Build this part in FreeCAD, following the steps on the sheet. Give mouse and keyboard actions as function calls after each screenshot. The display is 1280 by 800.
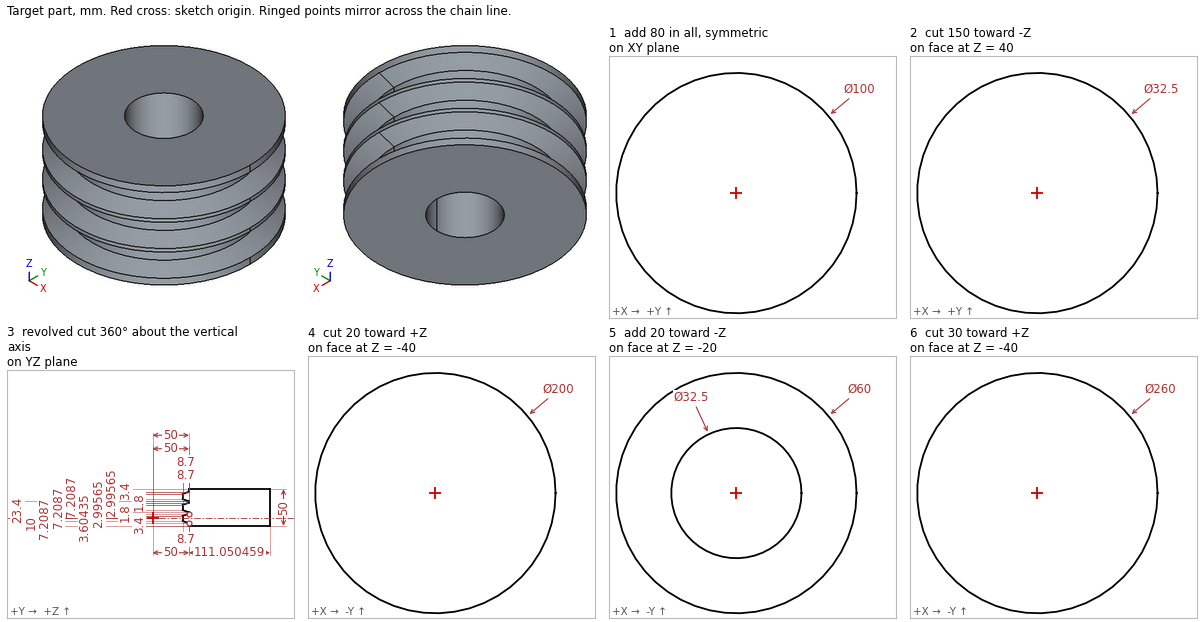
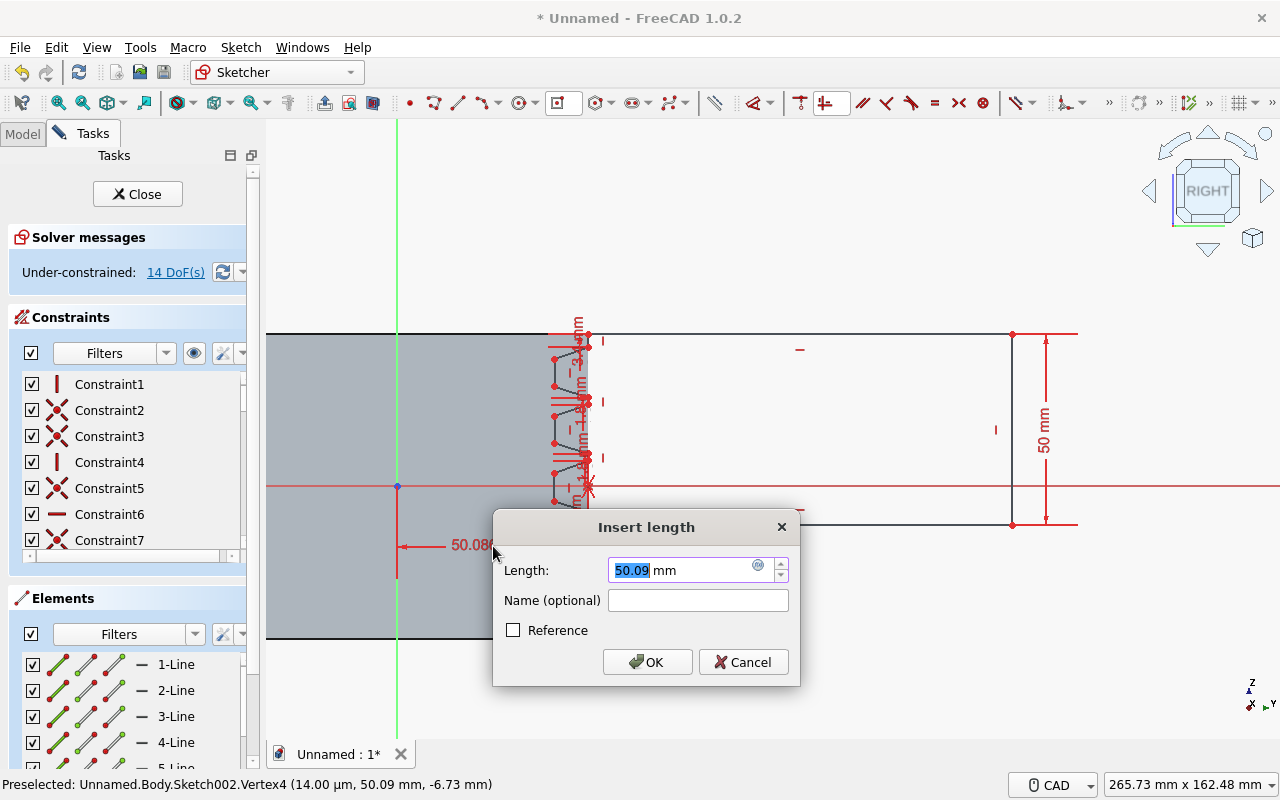
text(50)
key(Return)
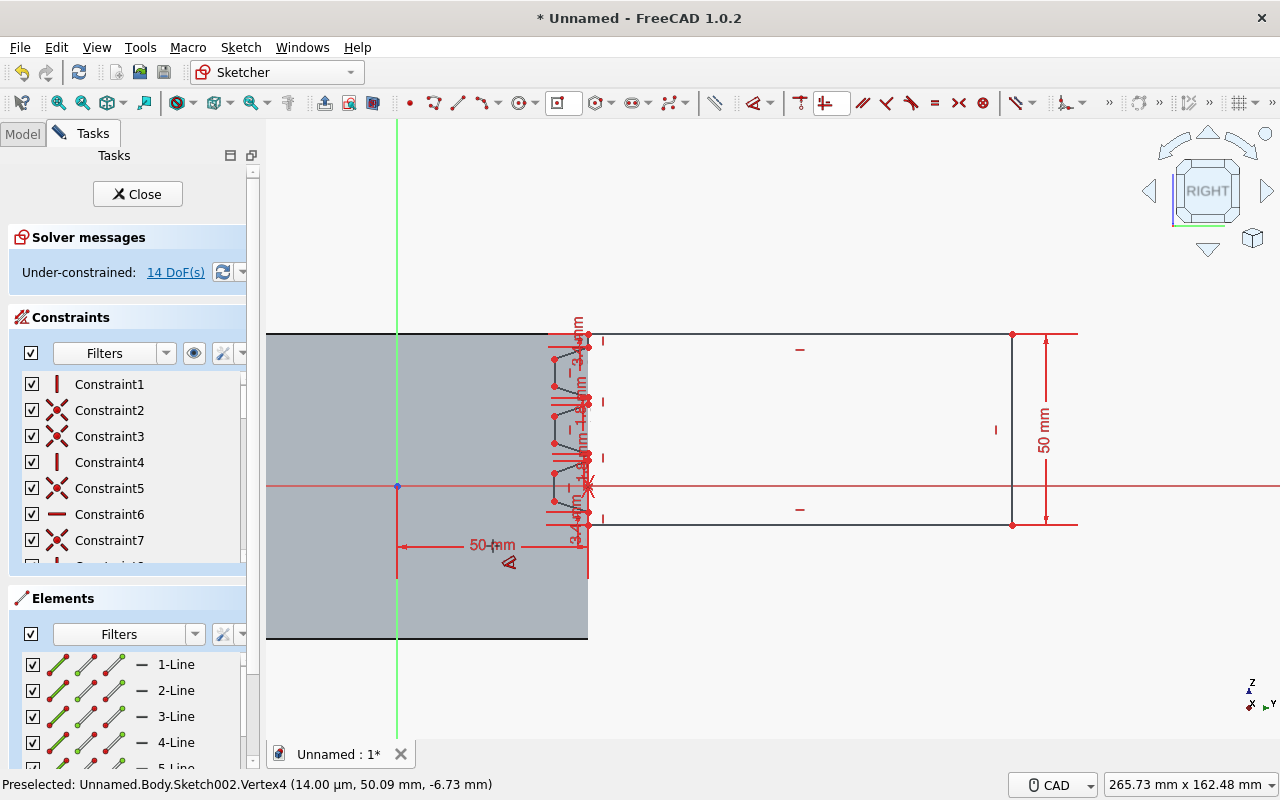
click(588, 525)
click(363, 506)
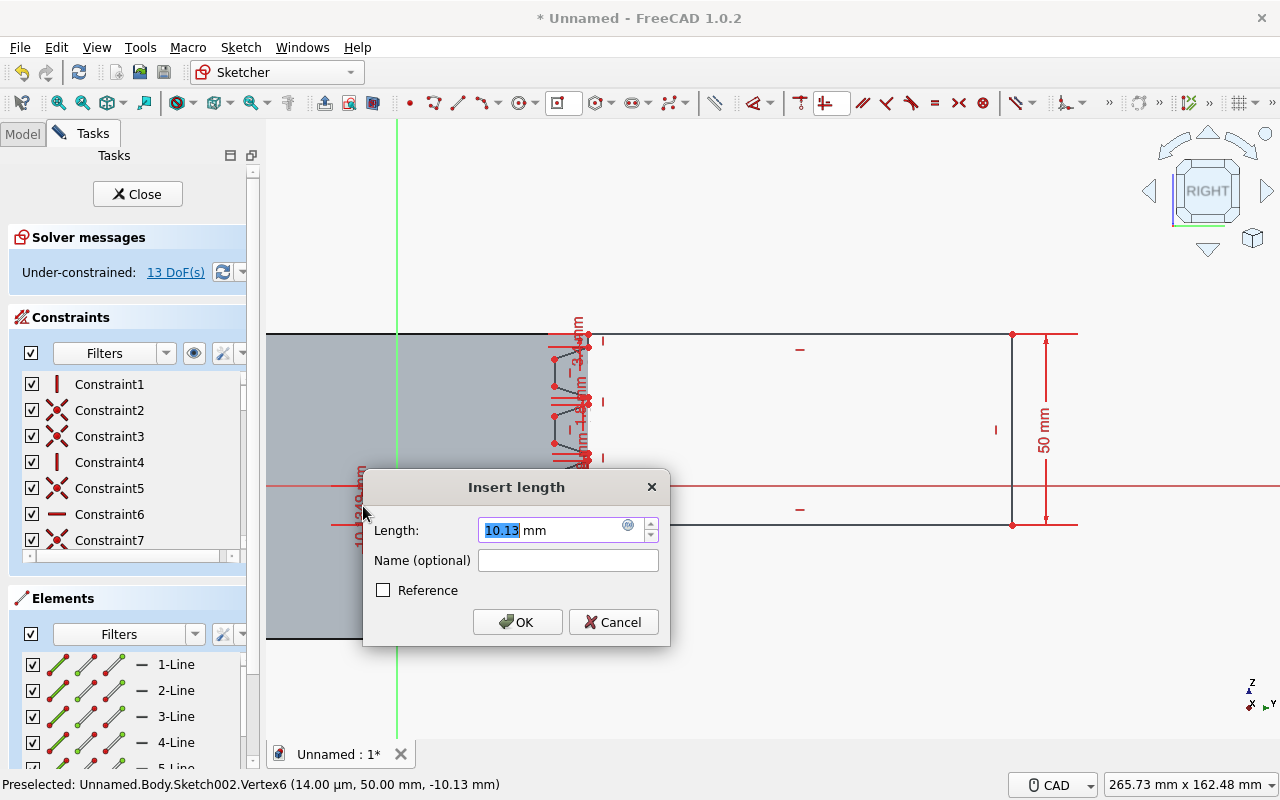
text(10)
key(Return)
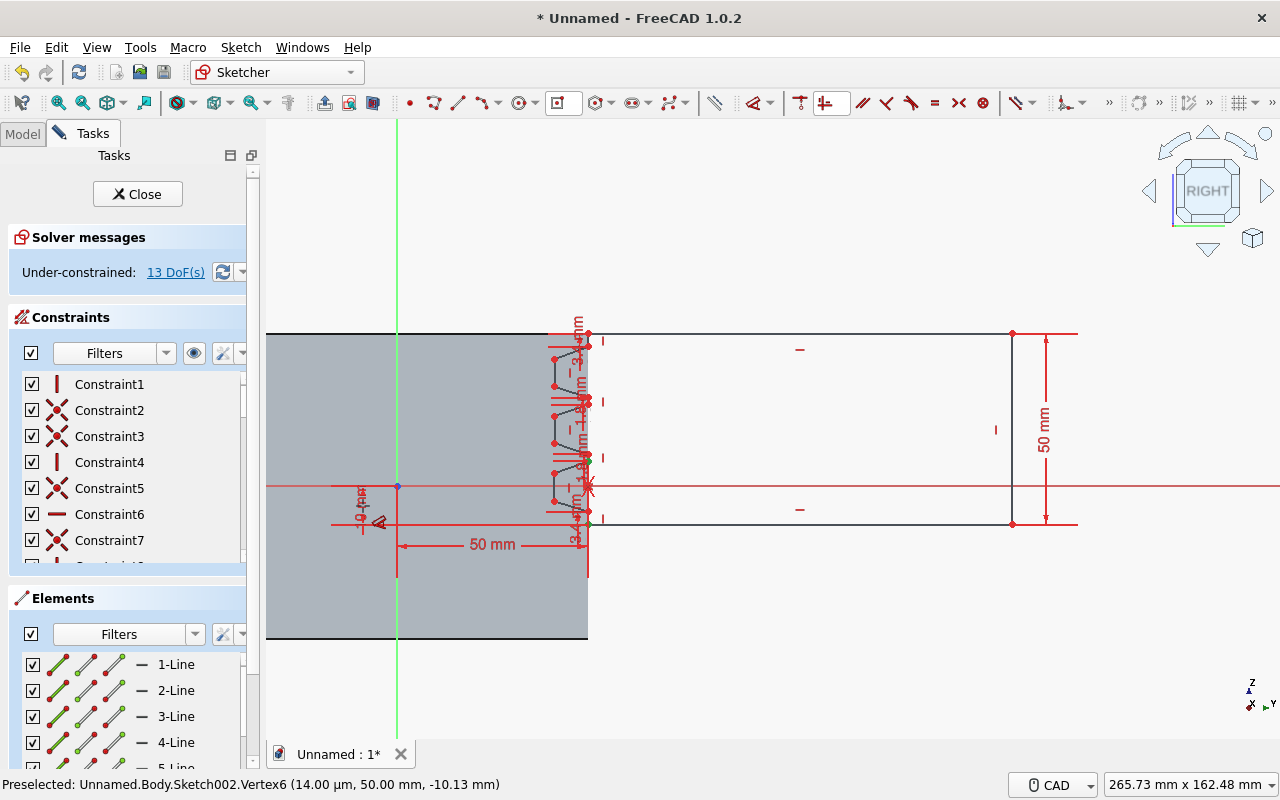
click(588, 334)
click(493, 300)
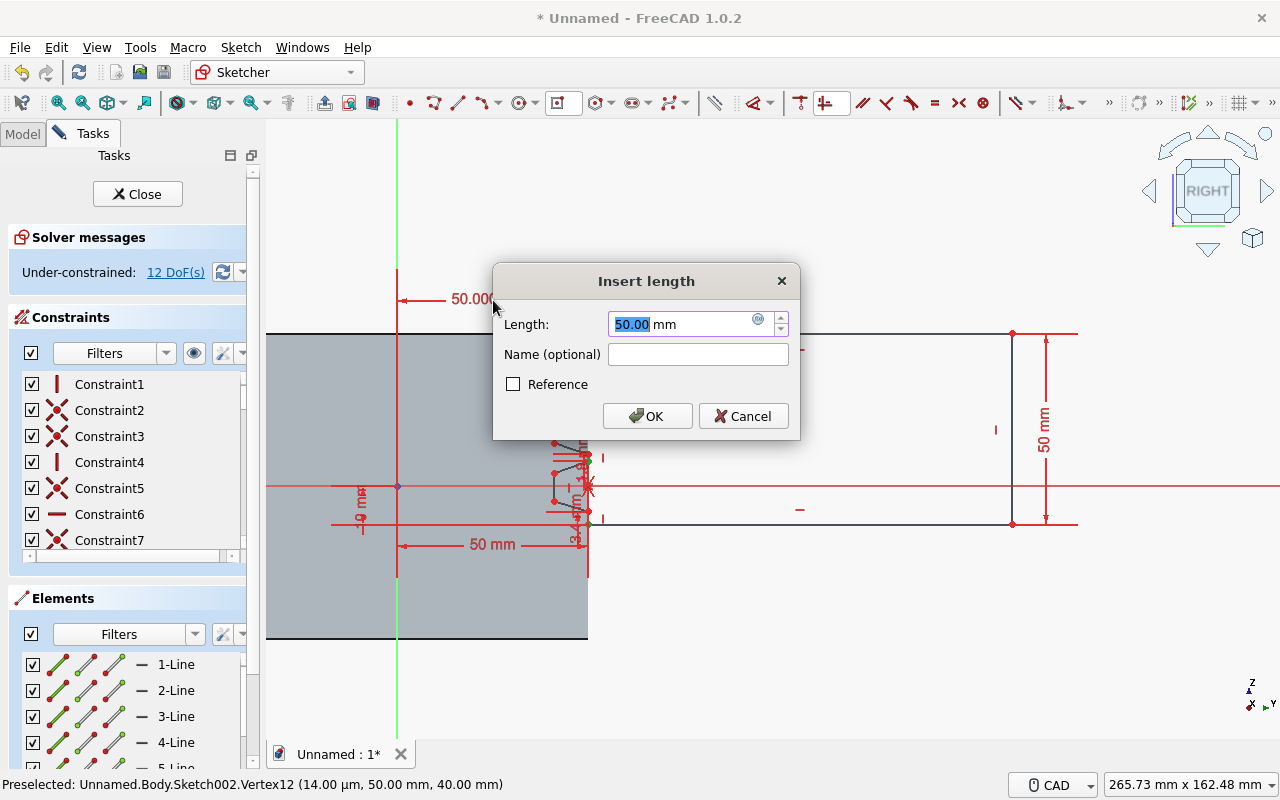
text(50)
key(Return)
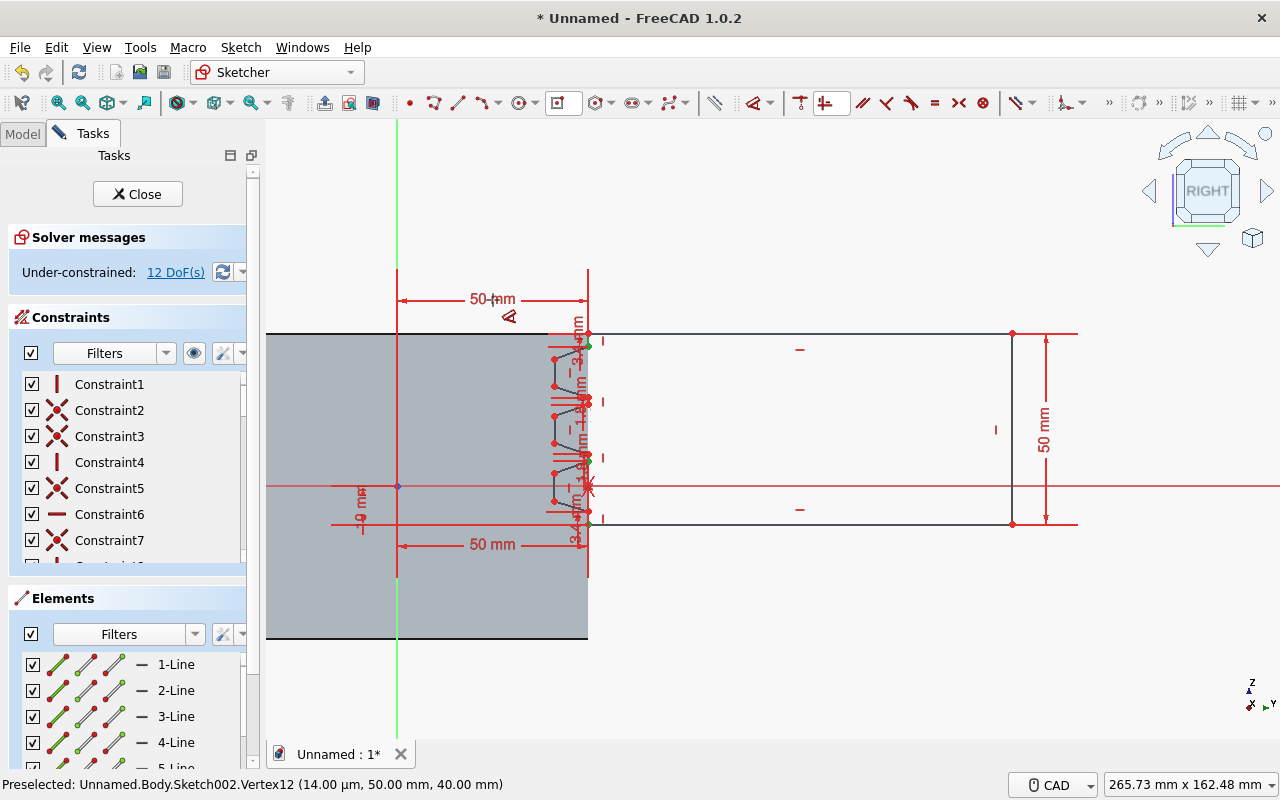
scroll(588, 398, up, 3)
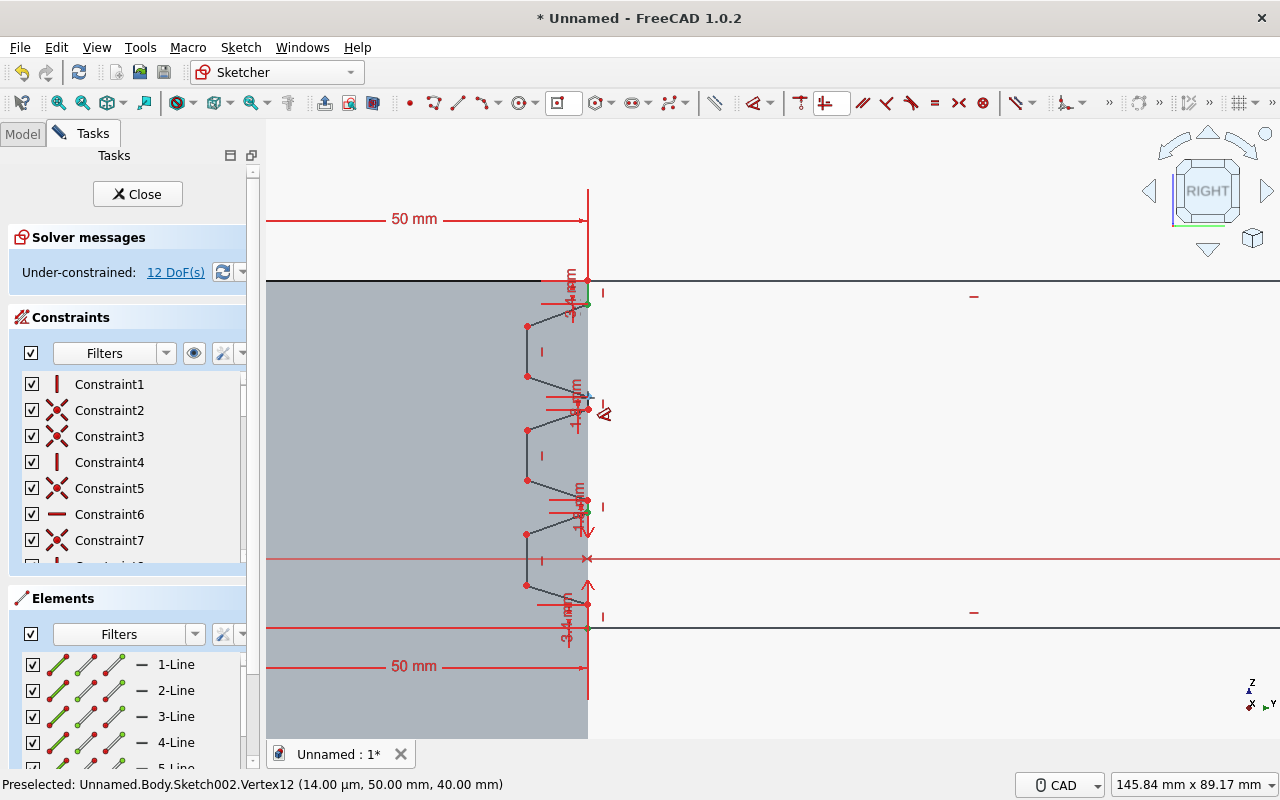
click(588, 397)
click(441, 593)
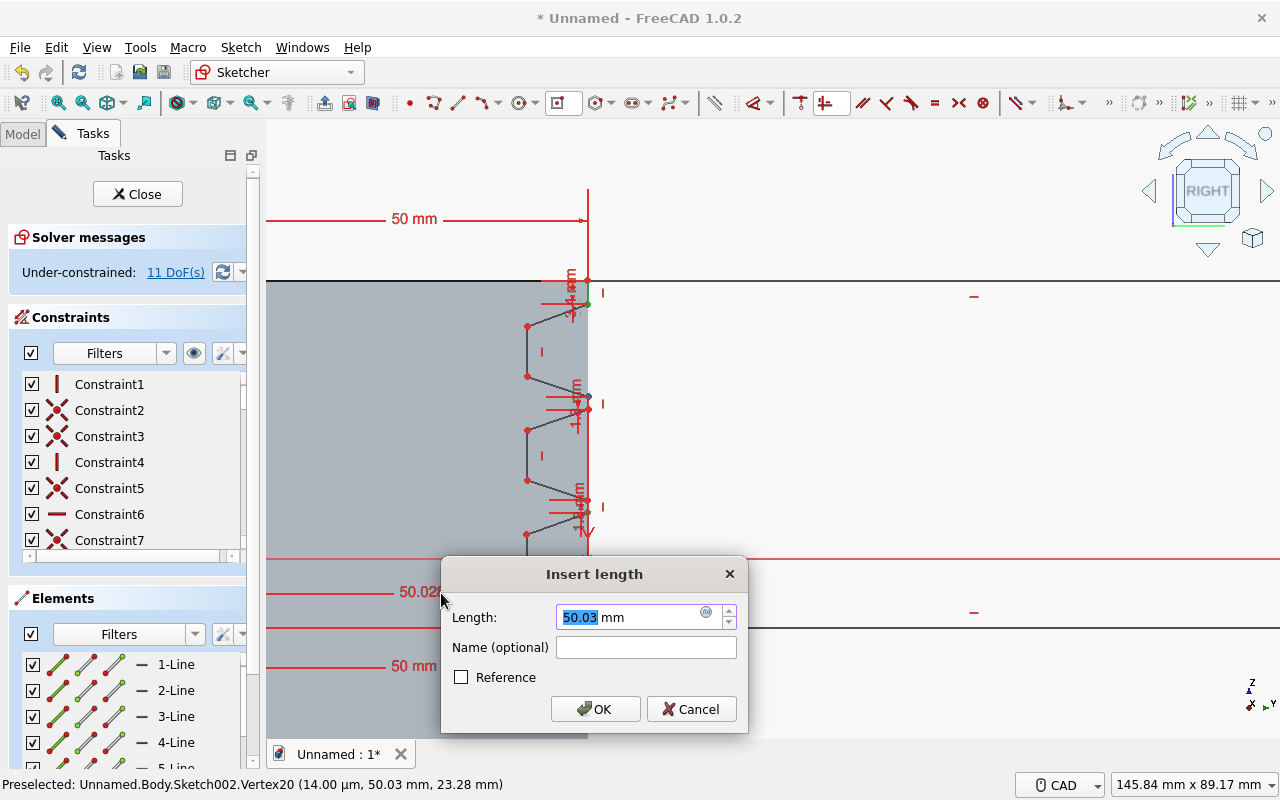
text(50)
key(Return)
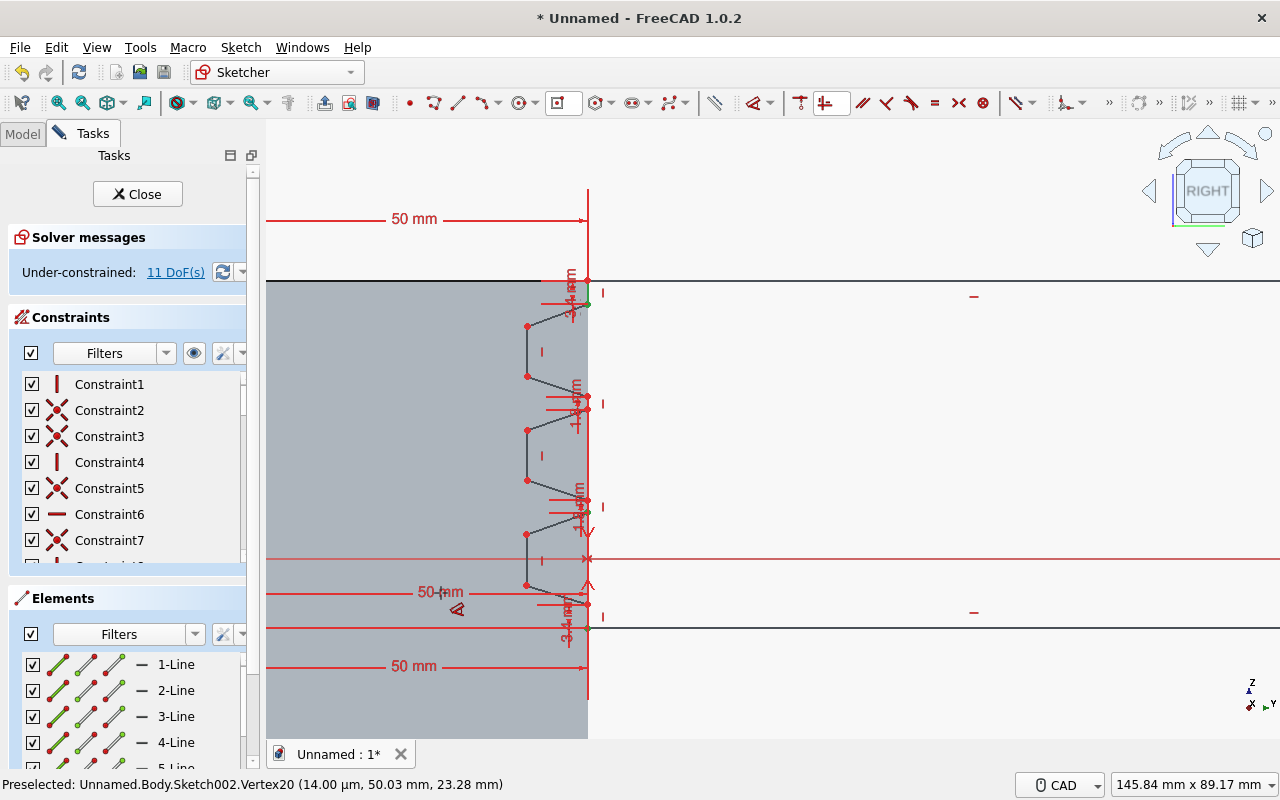
click(545, 592)
click(557, 639)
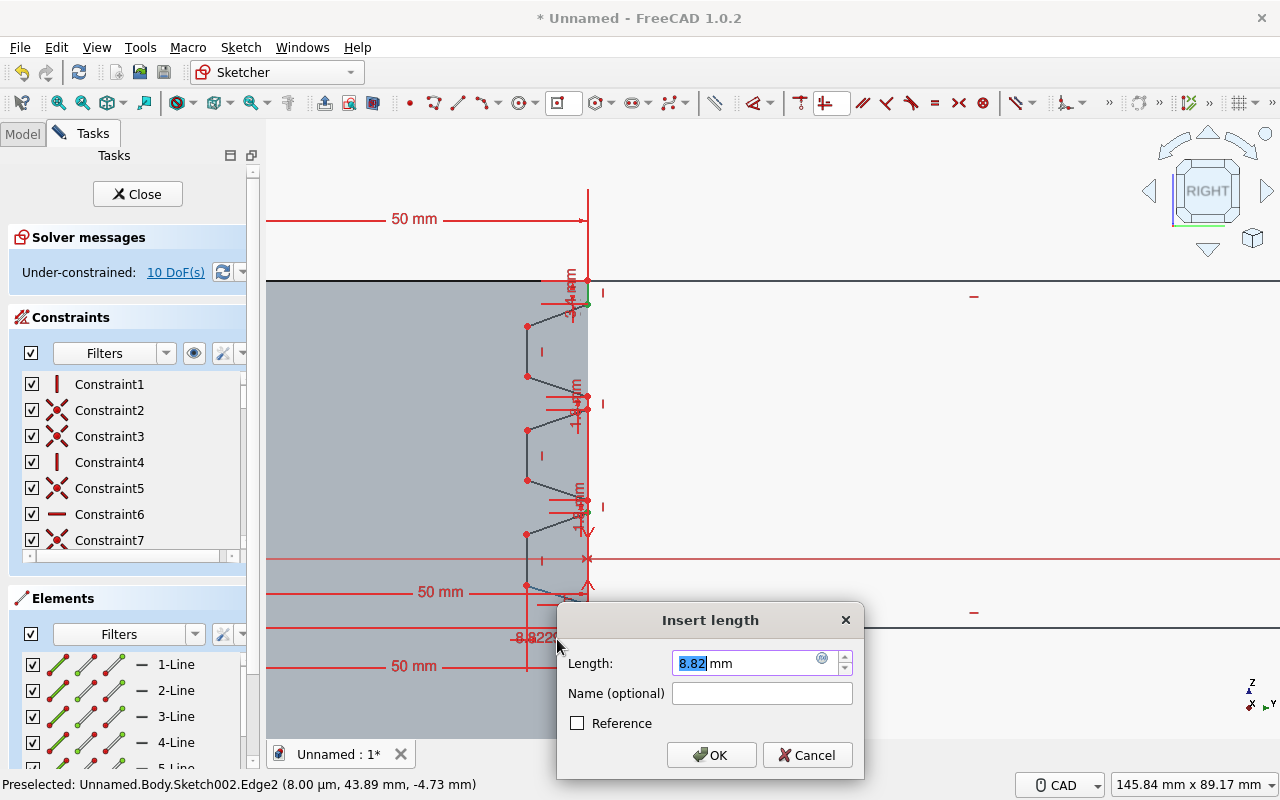
text(8.7)
key(Return)